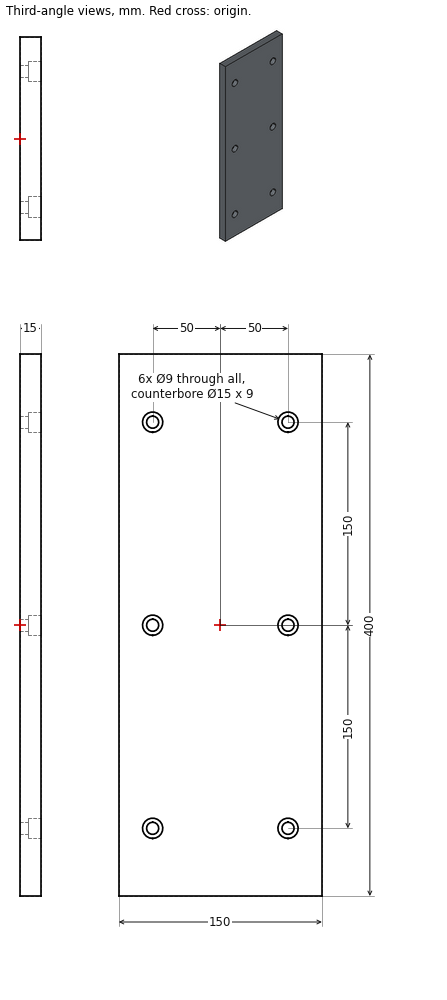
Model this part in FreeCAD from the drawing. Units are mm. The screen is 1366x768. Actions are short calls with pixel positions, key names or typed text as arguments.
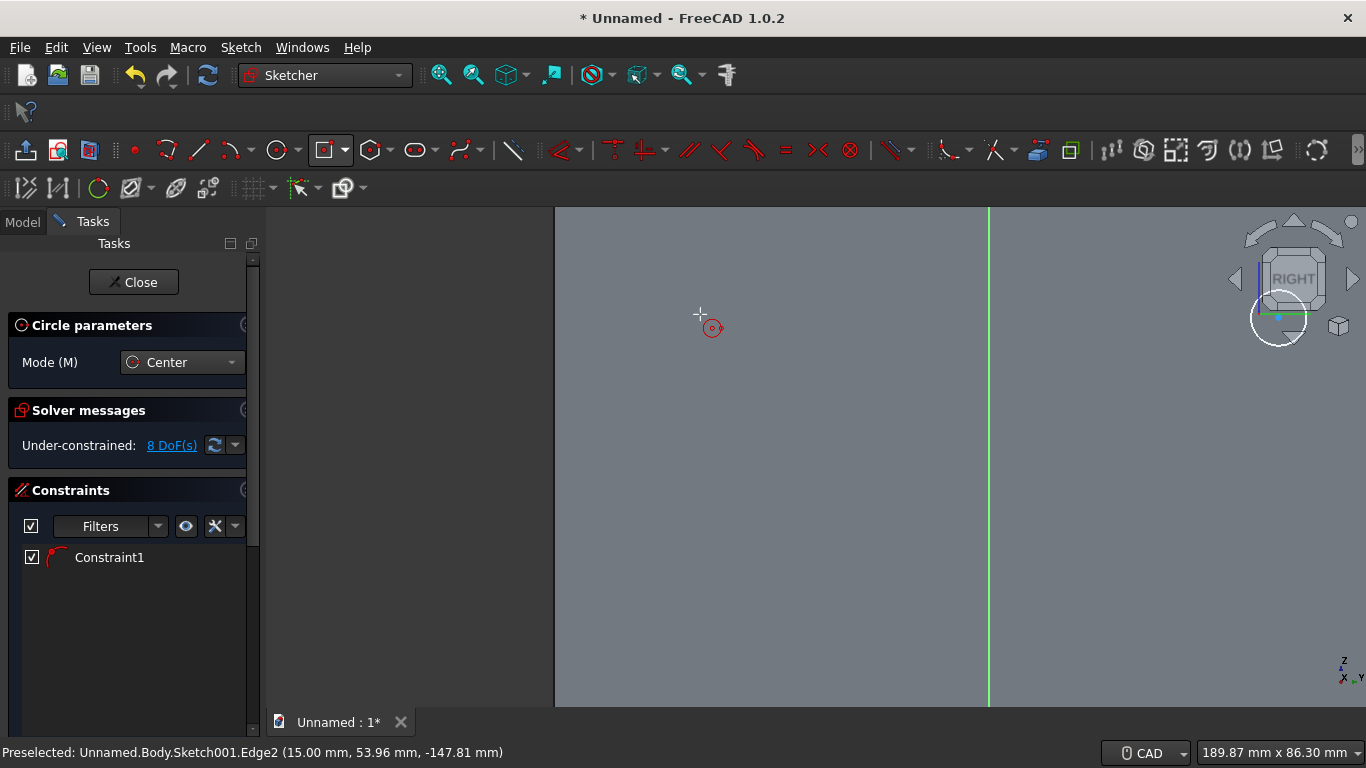
scroll(700, 313, down, 9)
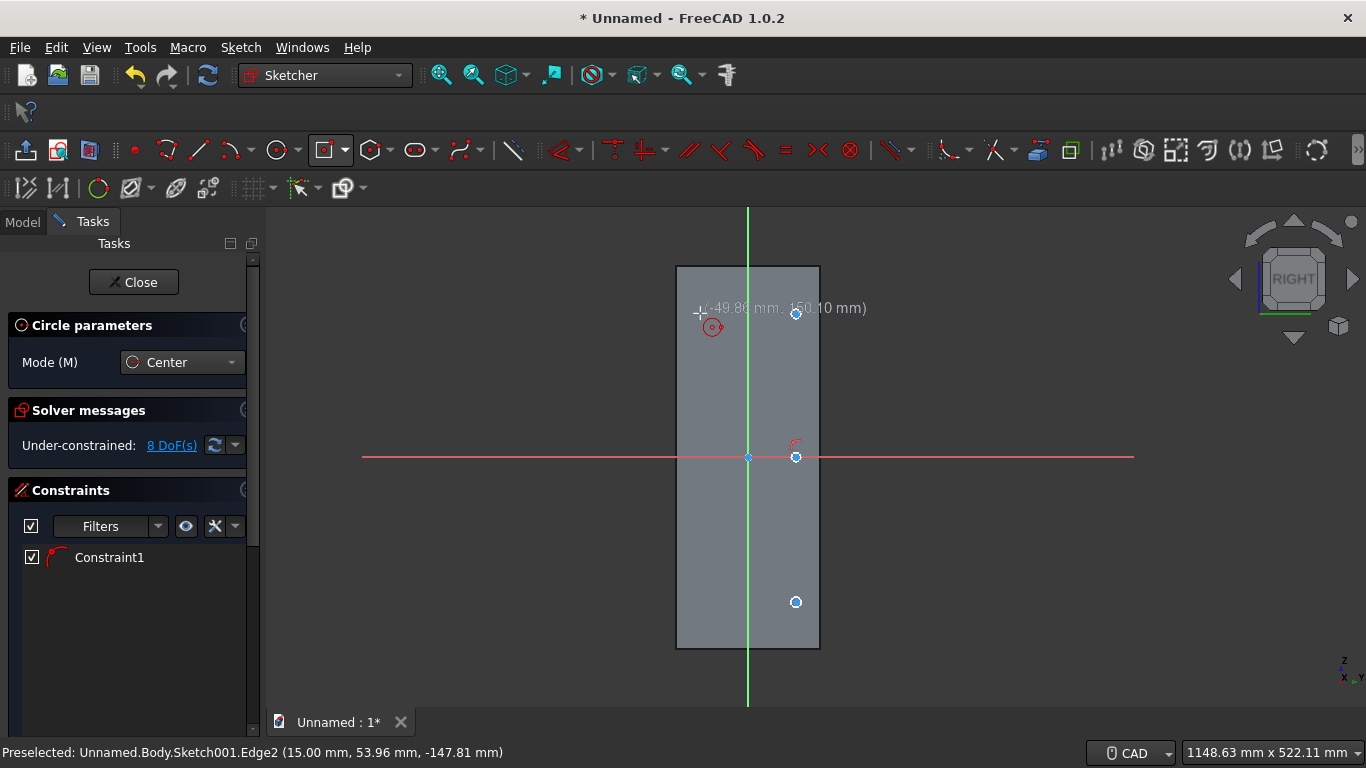
click(700, 313)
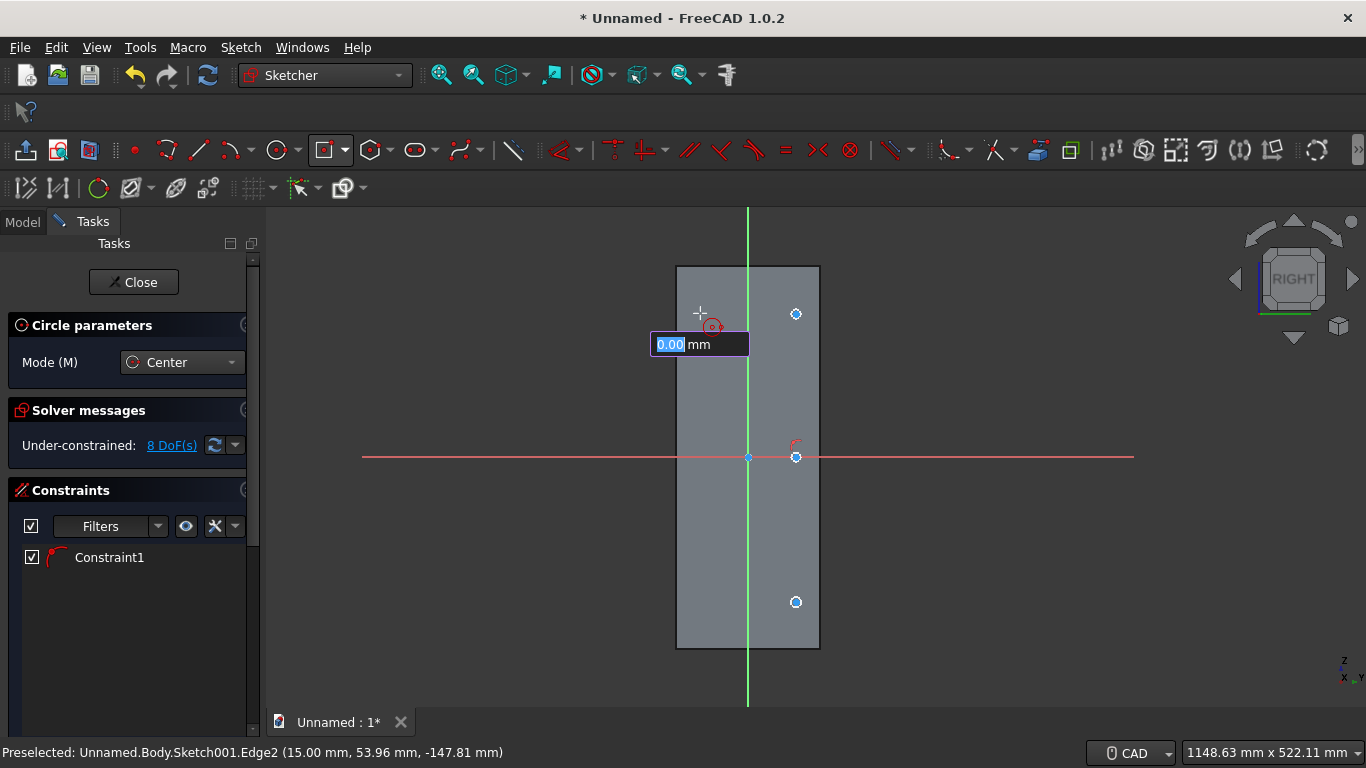
scroll(703, 310, up, 7)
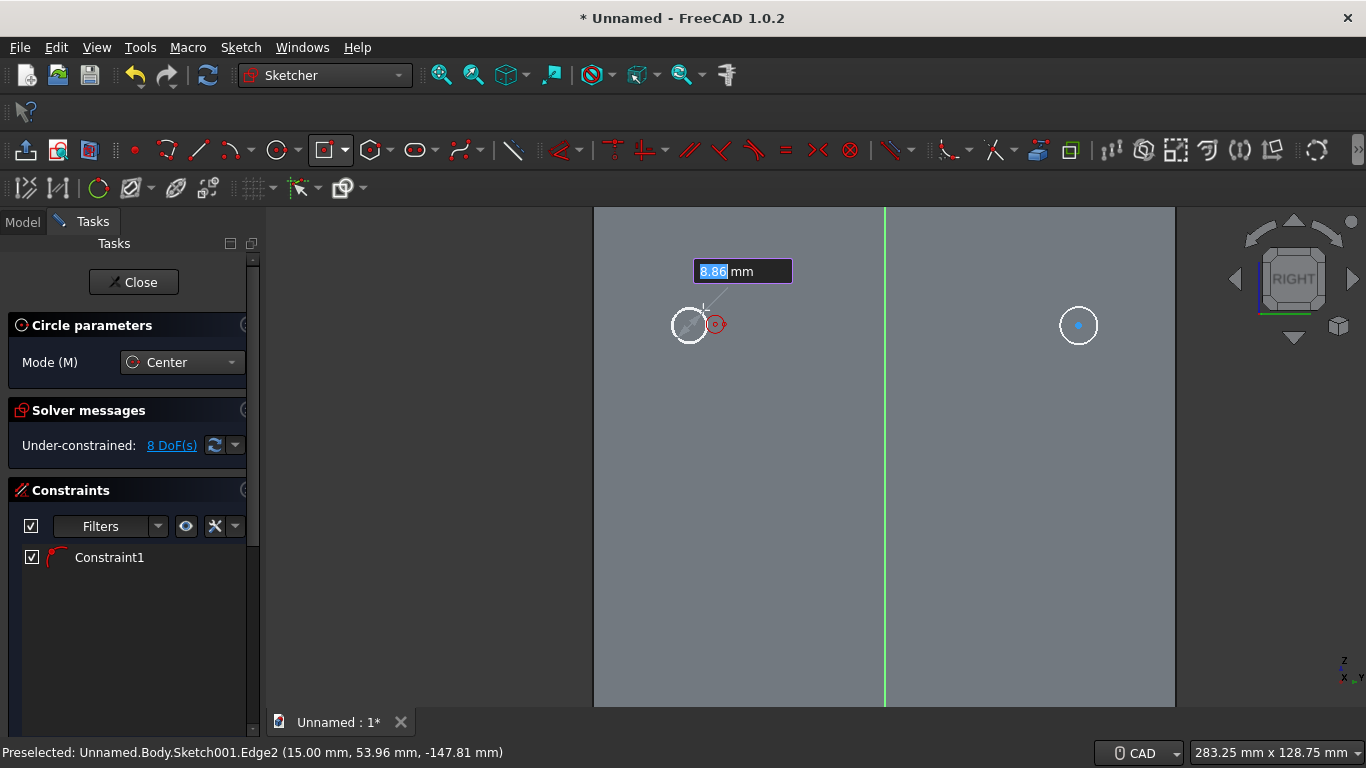
click(703, 311)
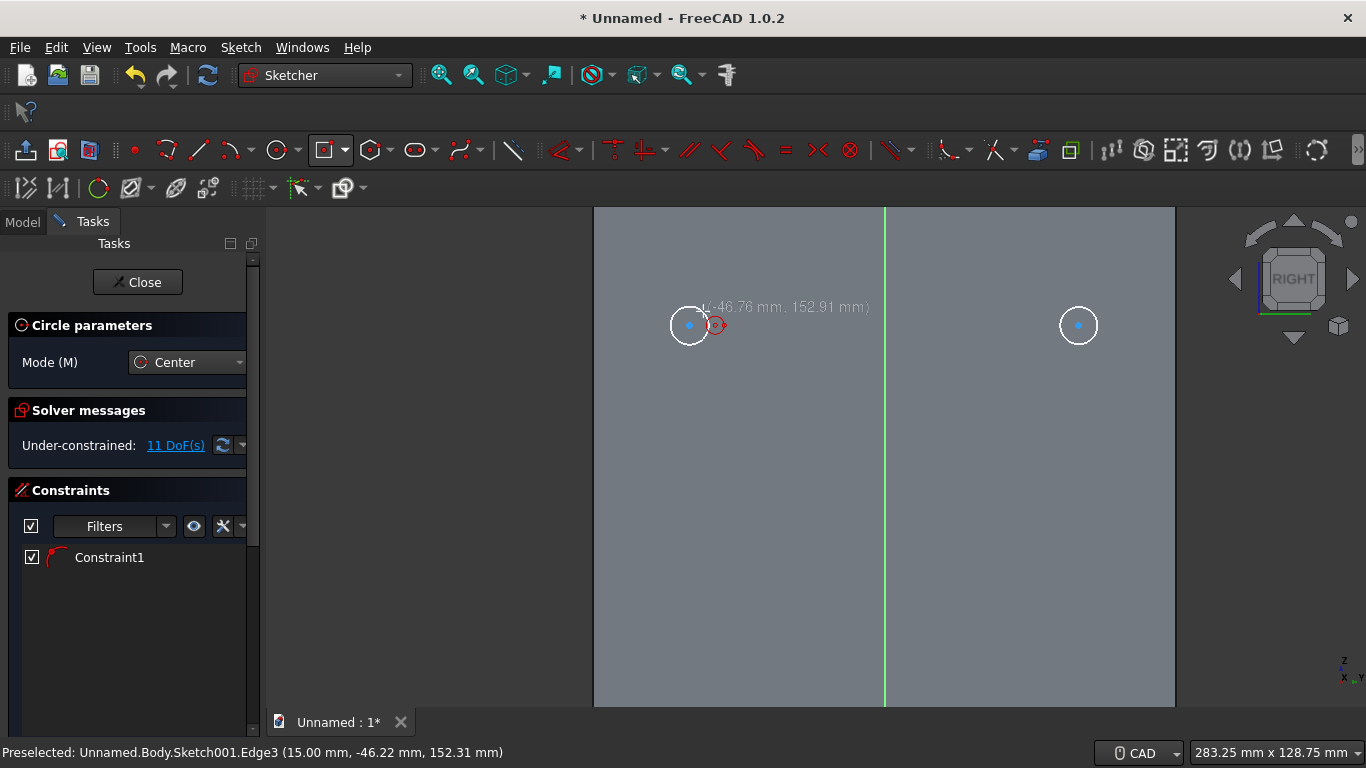
scroll(703, 310, down, 7)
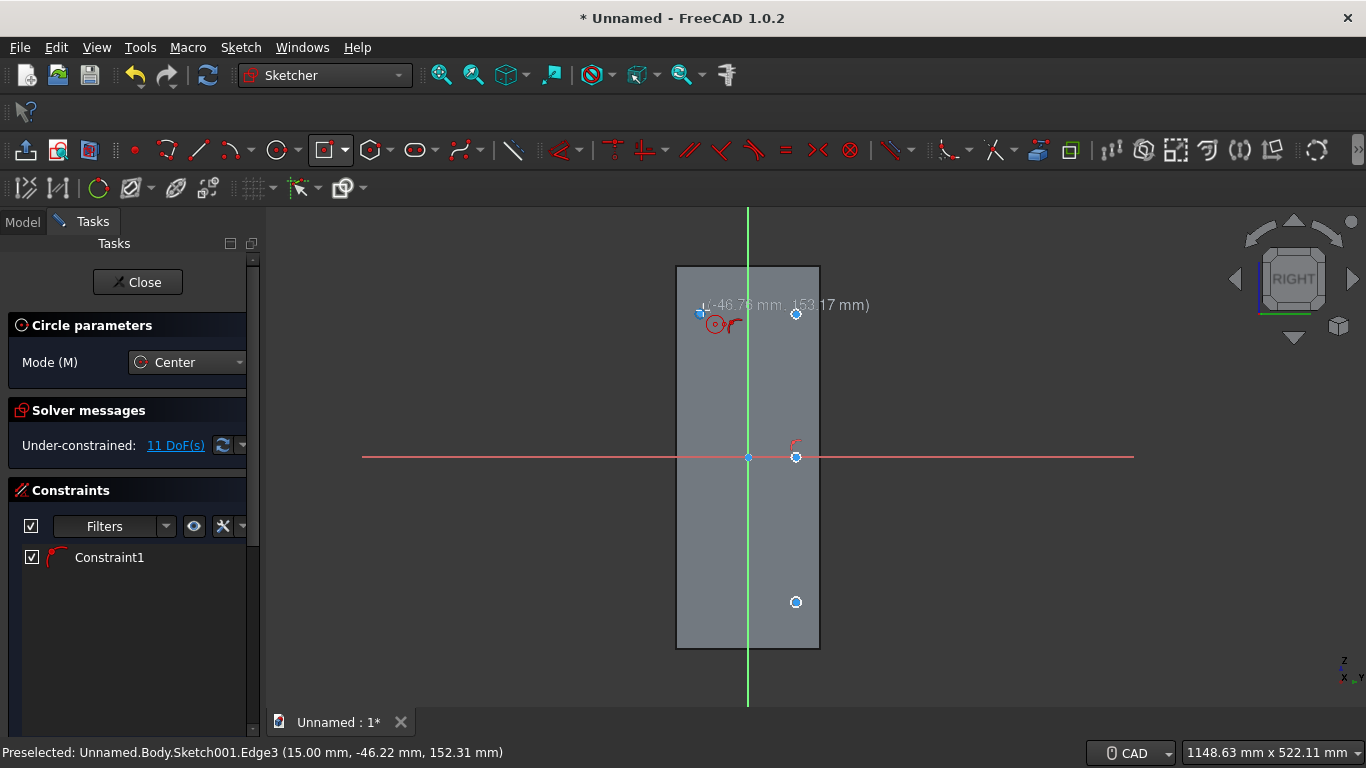
scroll(700, 457, up, 9)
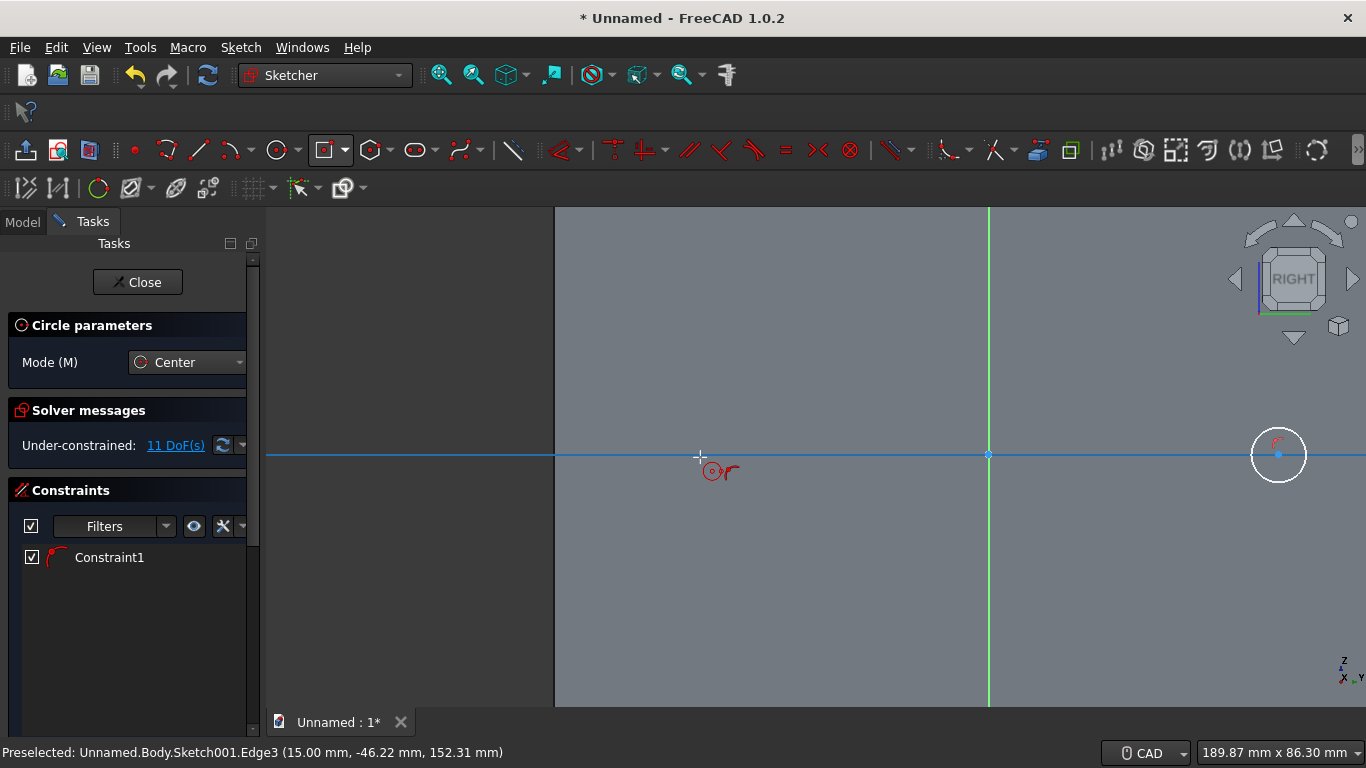
scroll(700, 457, down, 9)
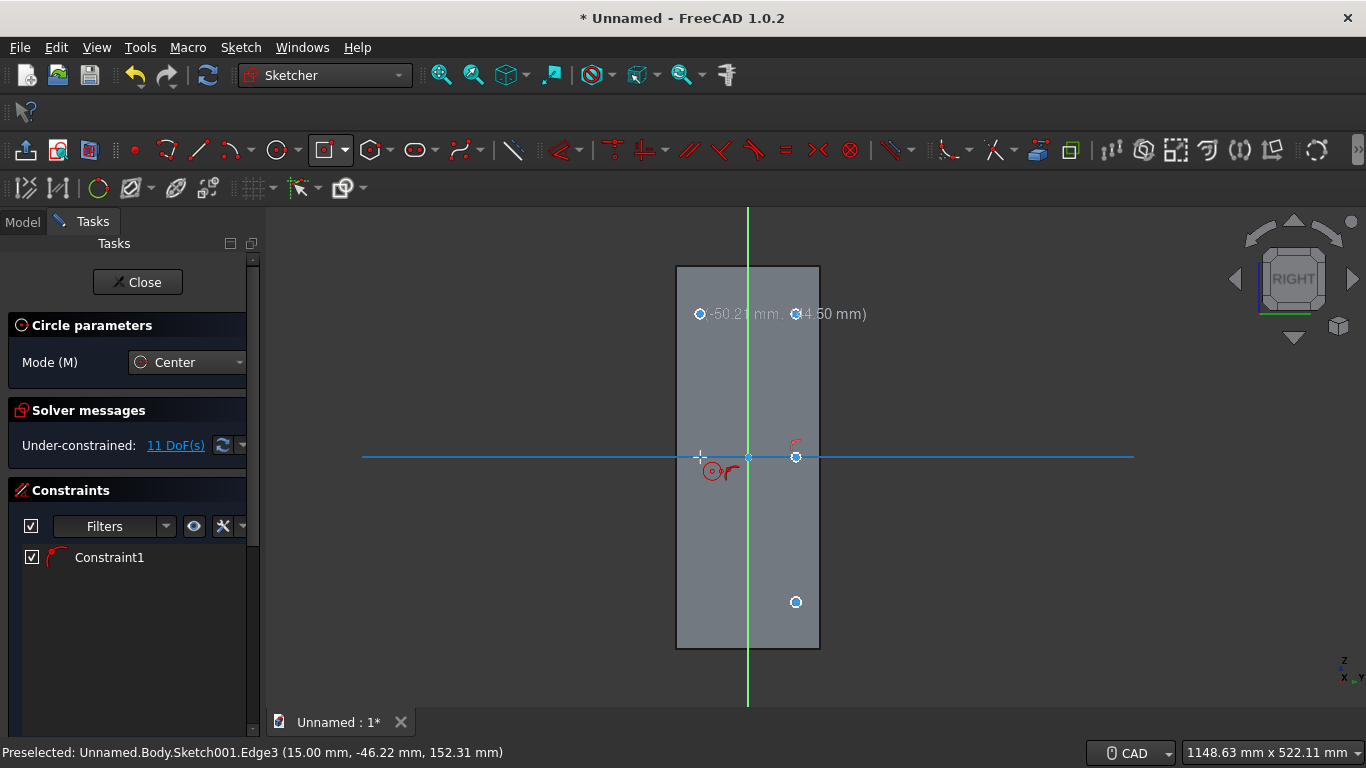
click(700, 457)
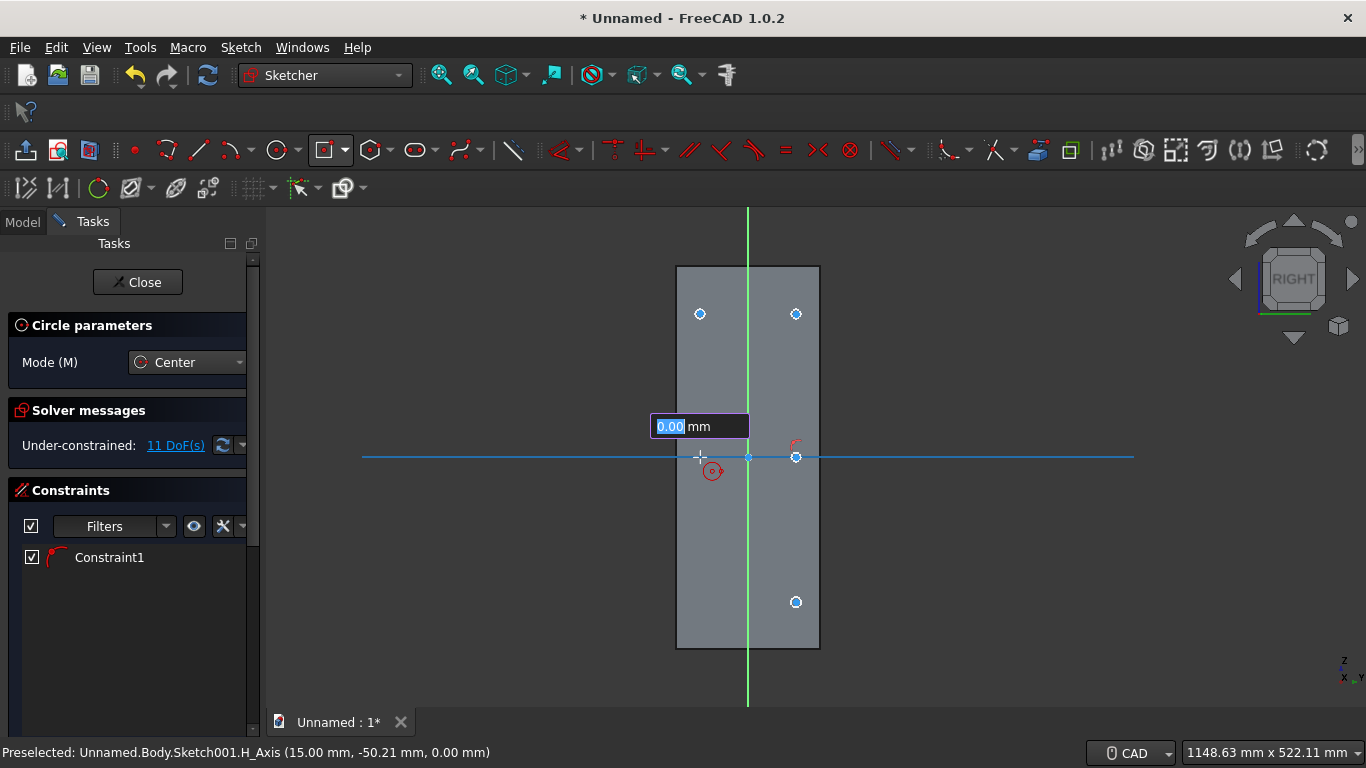
scroll(699, 461, up, 7)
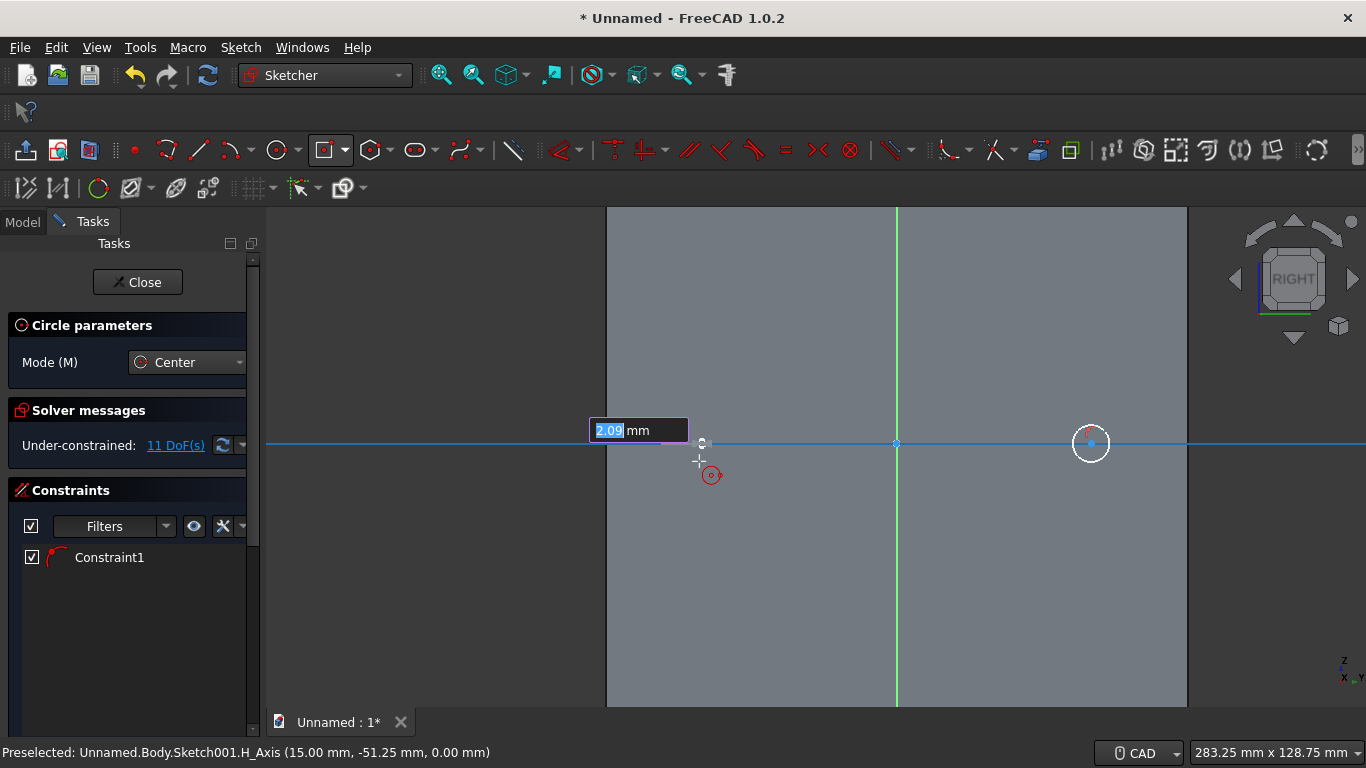
click(697, 460)